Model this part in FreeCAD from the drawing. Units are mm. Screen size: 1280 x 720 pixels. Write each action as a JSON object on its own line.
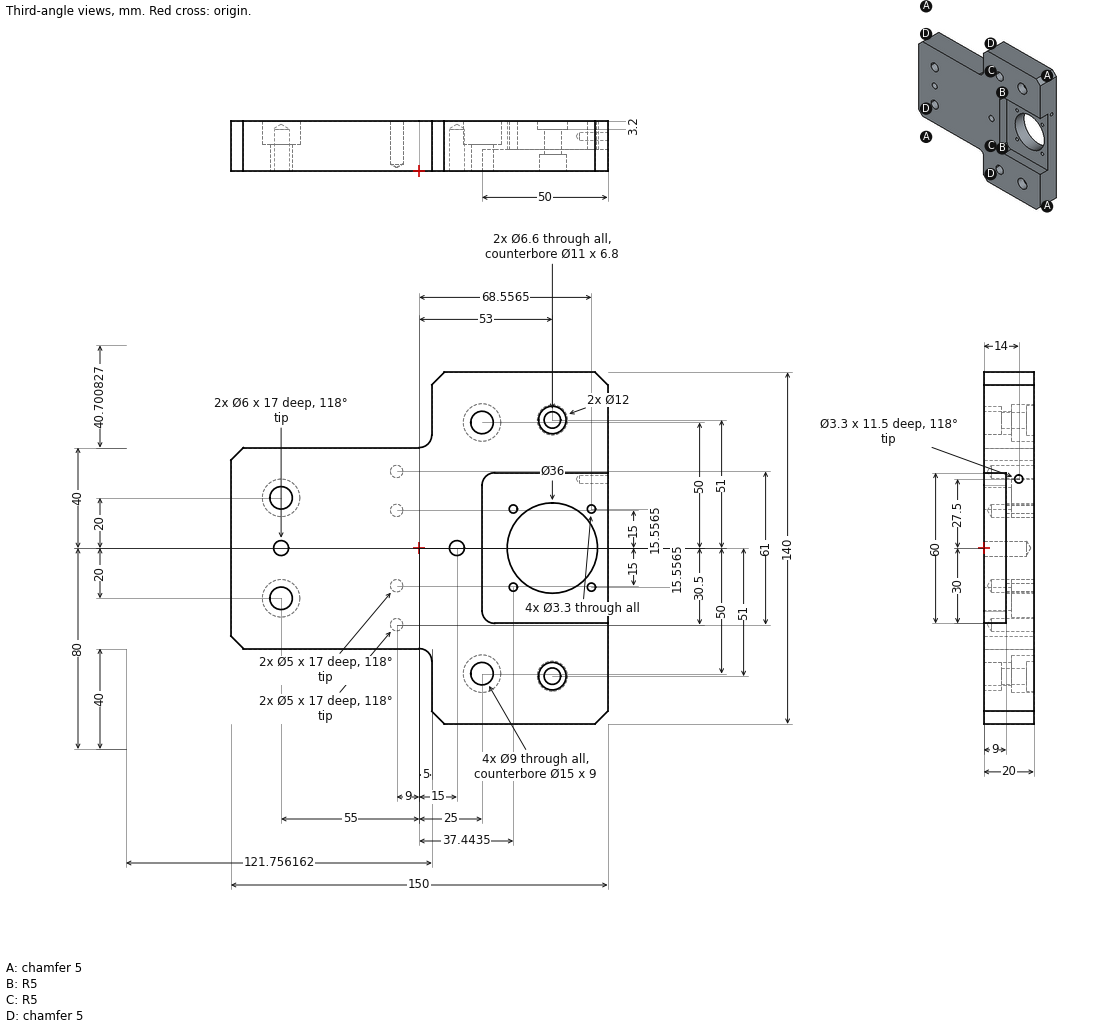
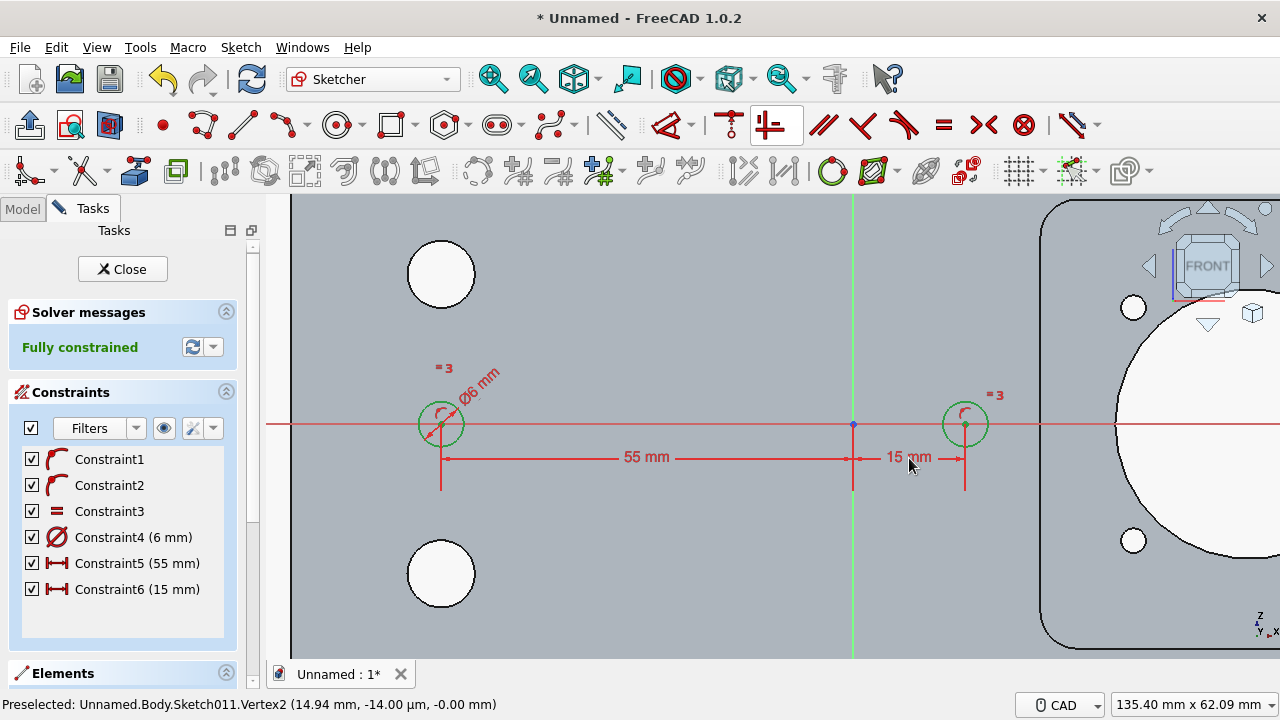
{"action": "left_click", "coordinate": [123, 269]}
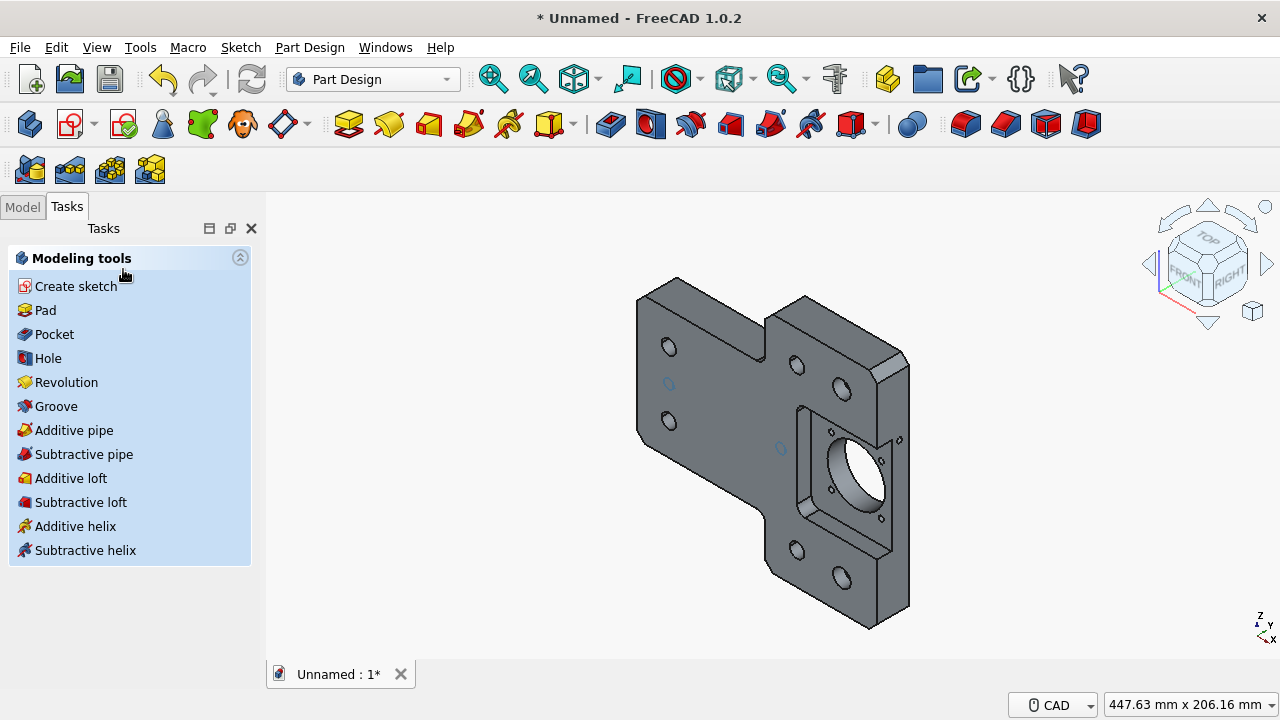
{"action": "left_click", "coordinate": [652, 124]}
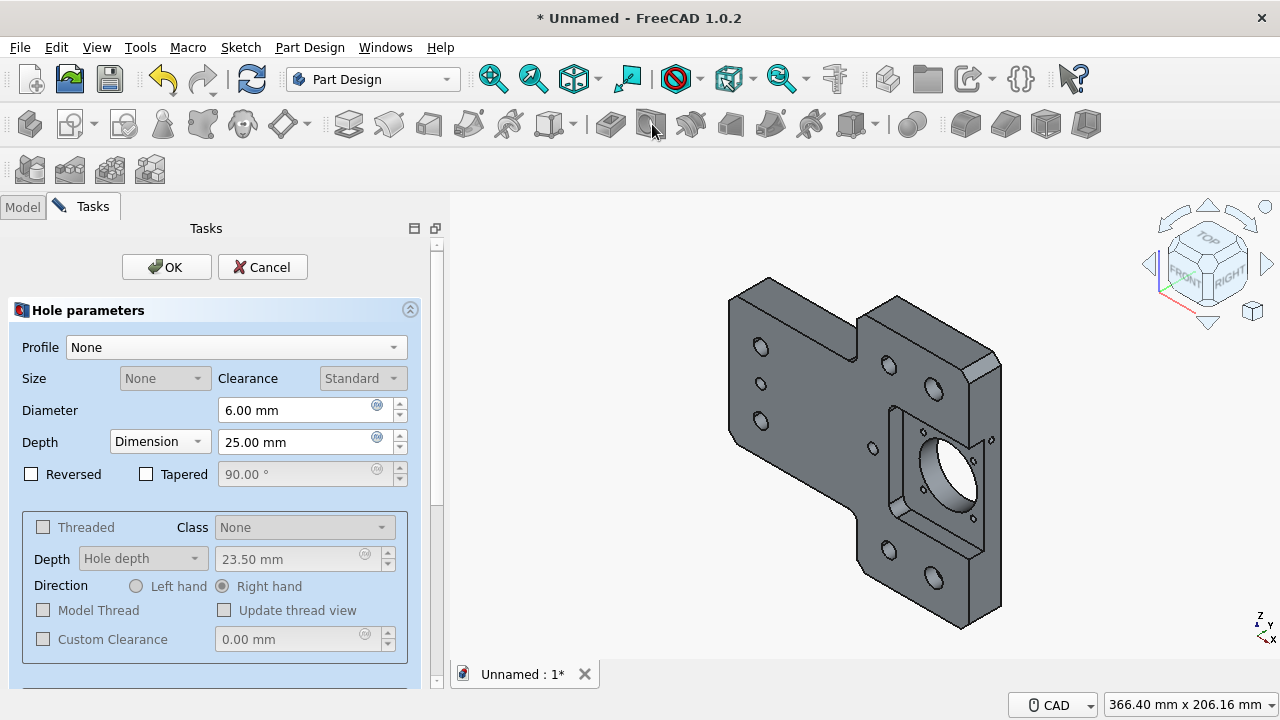
{"action": "triple_click", "coordinate": [305, 410]}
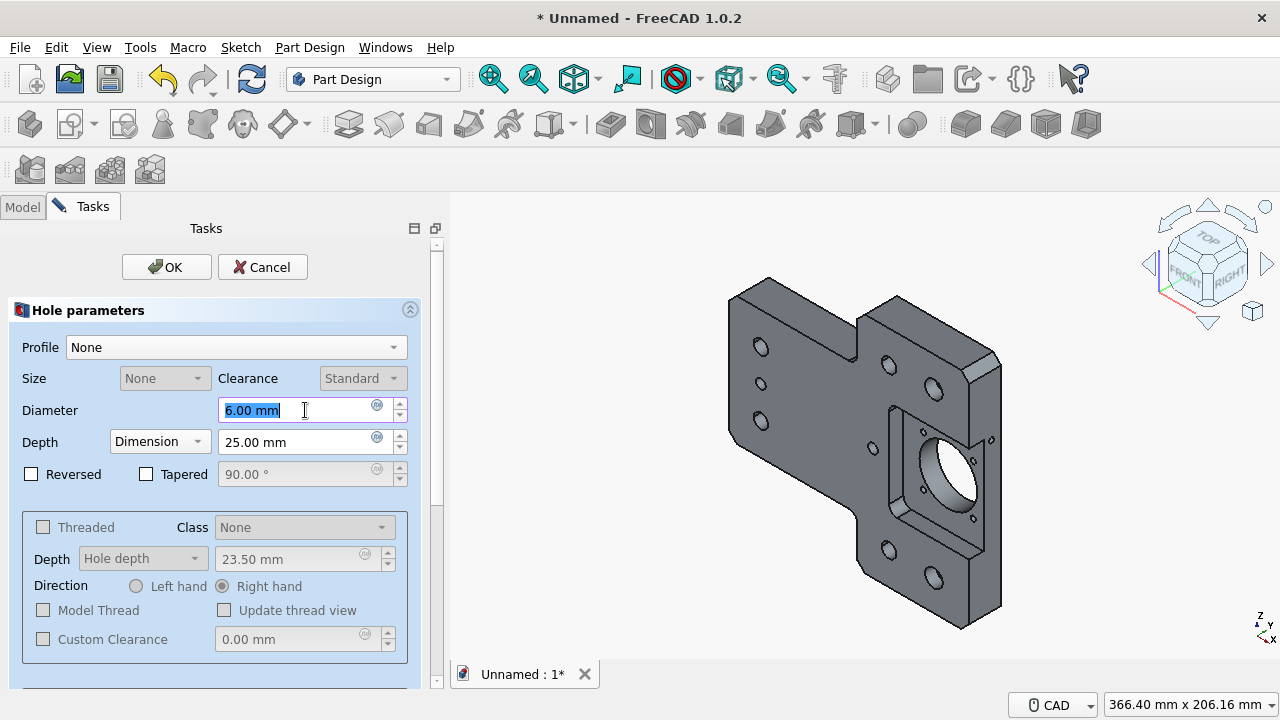
{"action": "type", "text": "6"}
{"action": "key", "text": "Tab"}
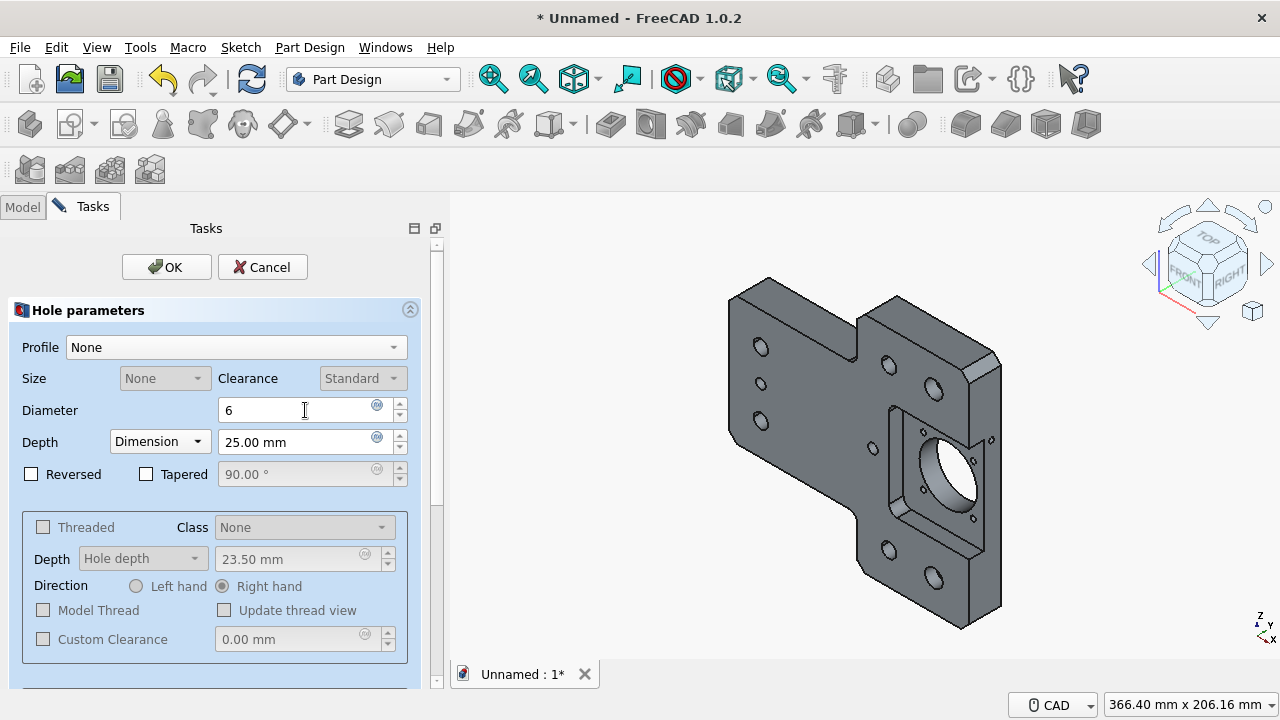
{"action": "triple_click", "coordinate": [305, 442]}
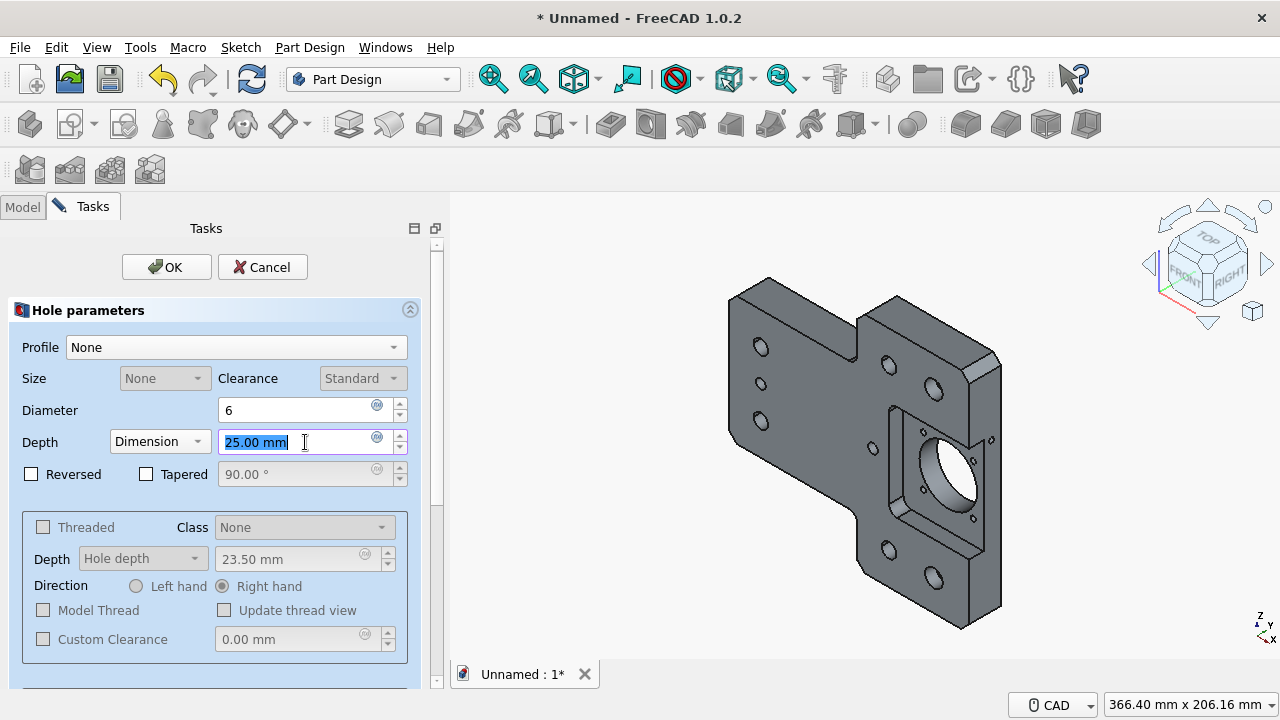
{"action": "type", "text": "17"}
{"action": "key", "text": "Tab"}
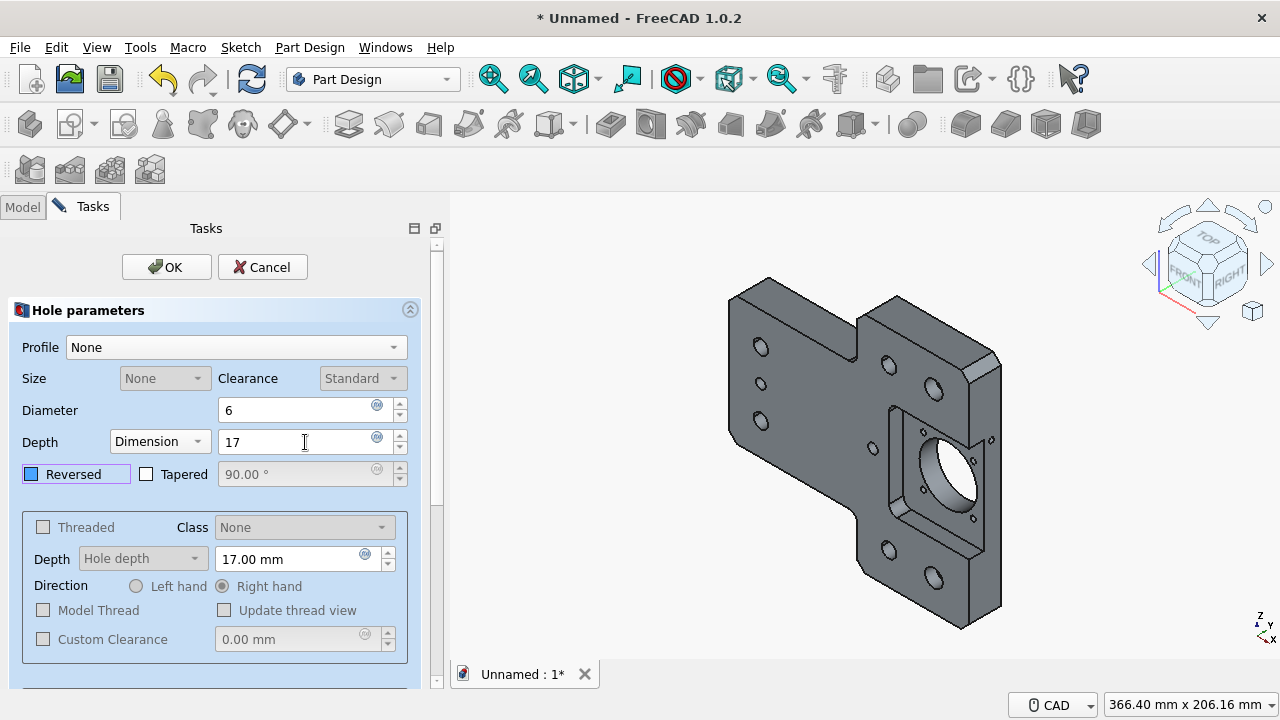
{"action": "left_click", "coordinate": [167, 267]}